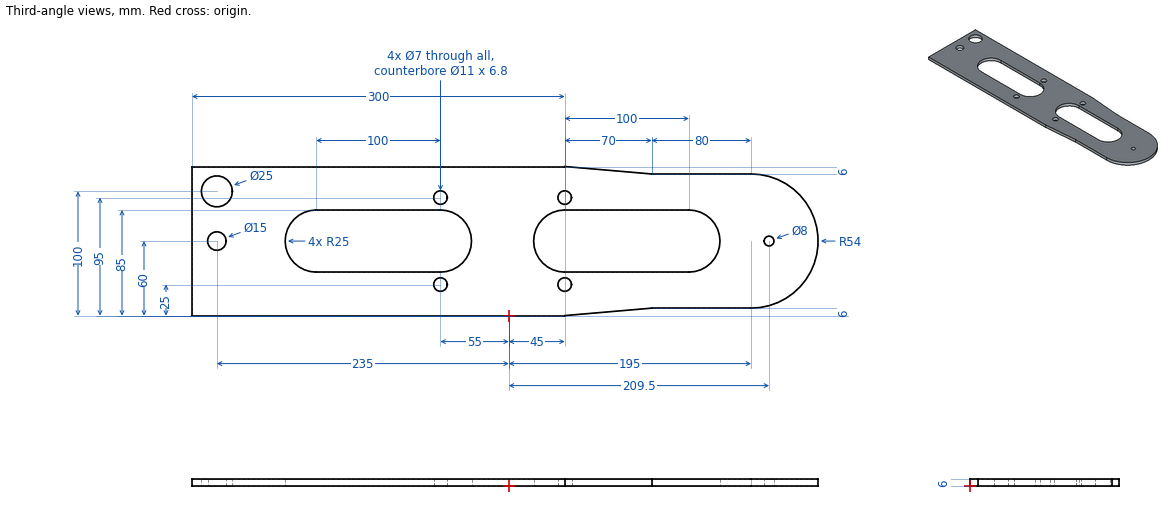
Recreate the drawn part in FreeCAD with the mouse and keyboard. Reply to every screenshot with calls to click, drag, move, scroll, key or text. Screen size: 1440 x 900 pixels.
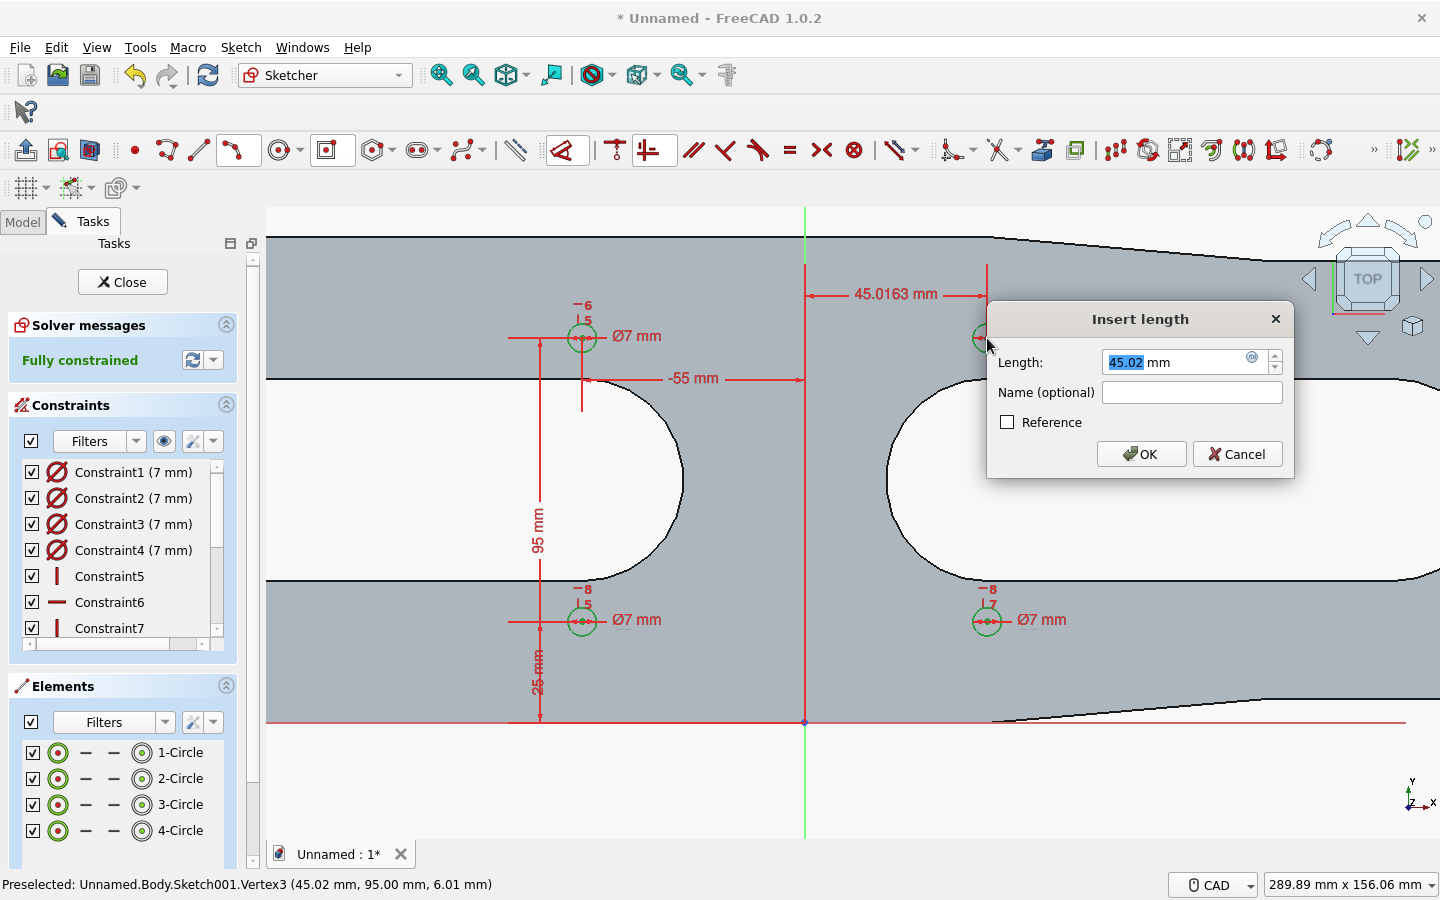
text(45)
key(Return)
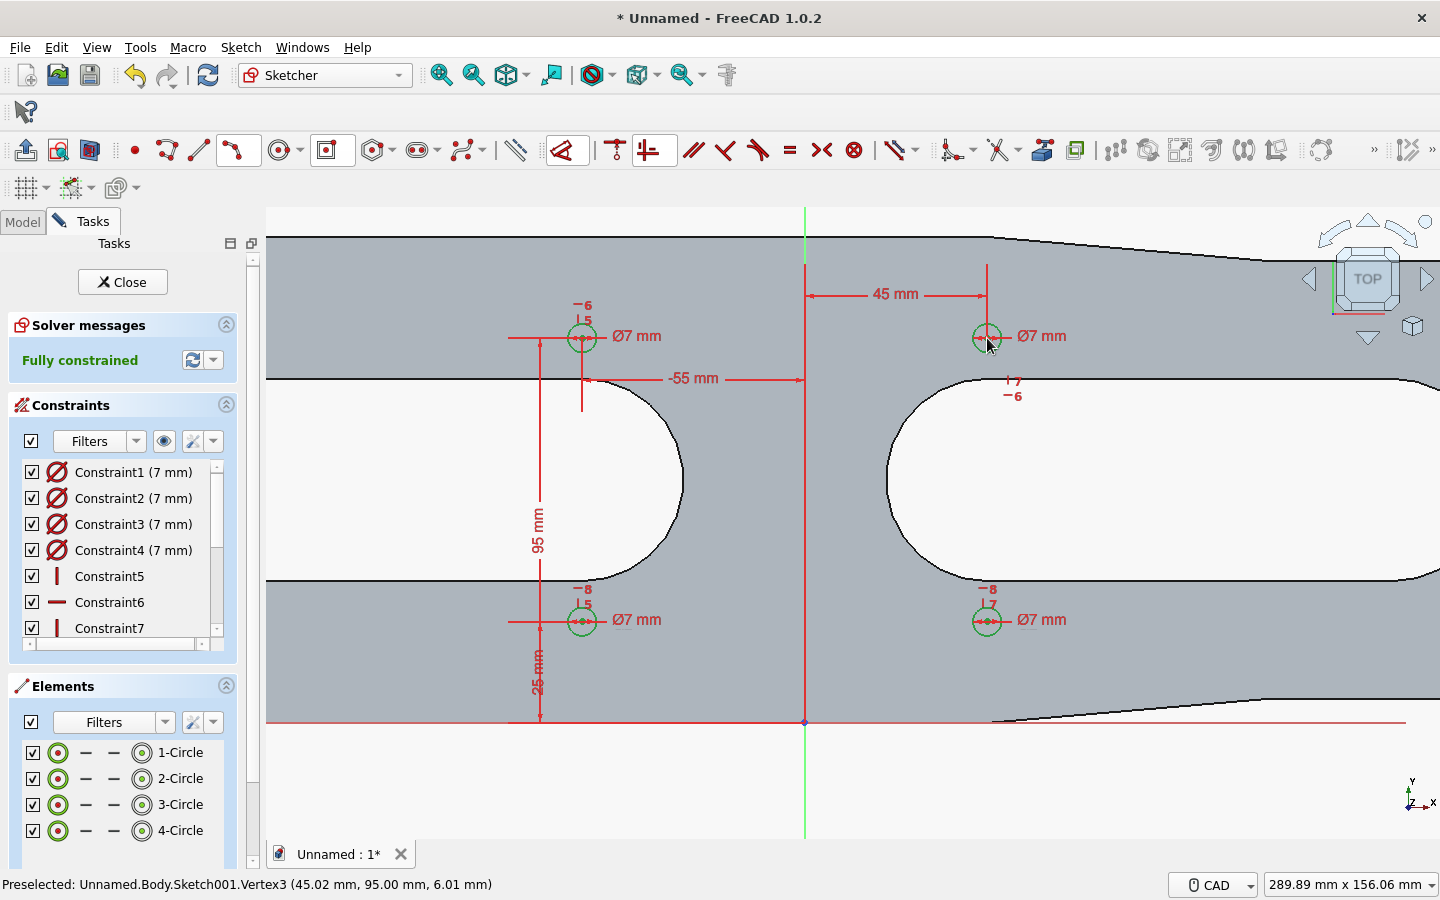
click(123, 282)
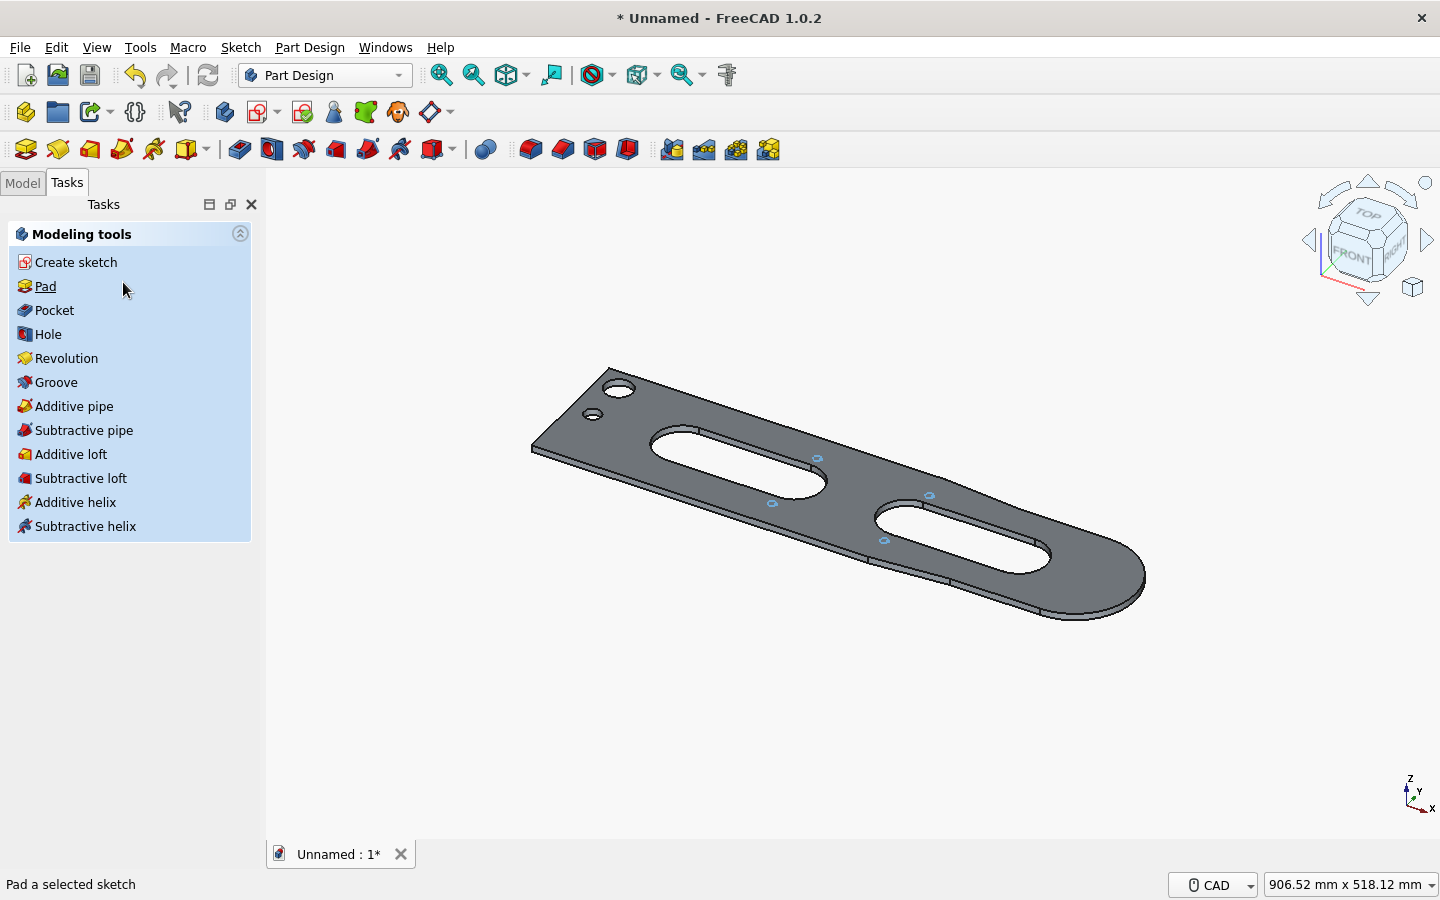
click(272, 150)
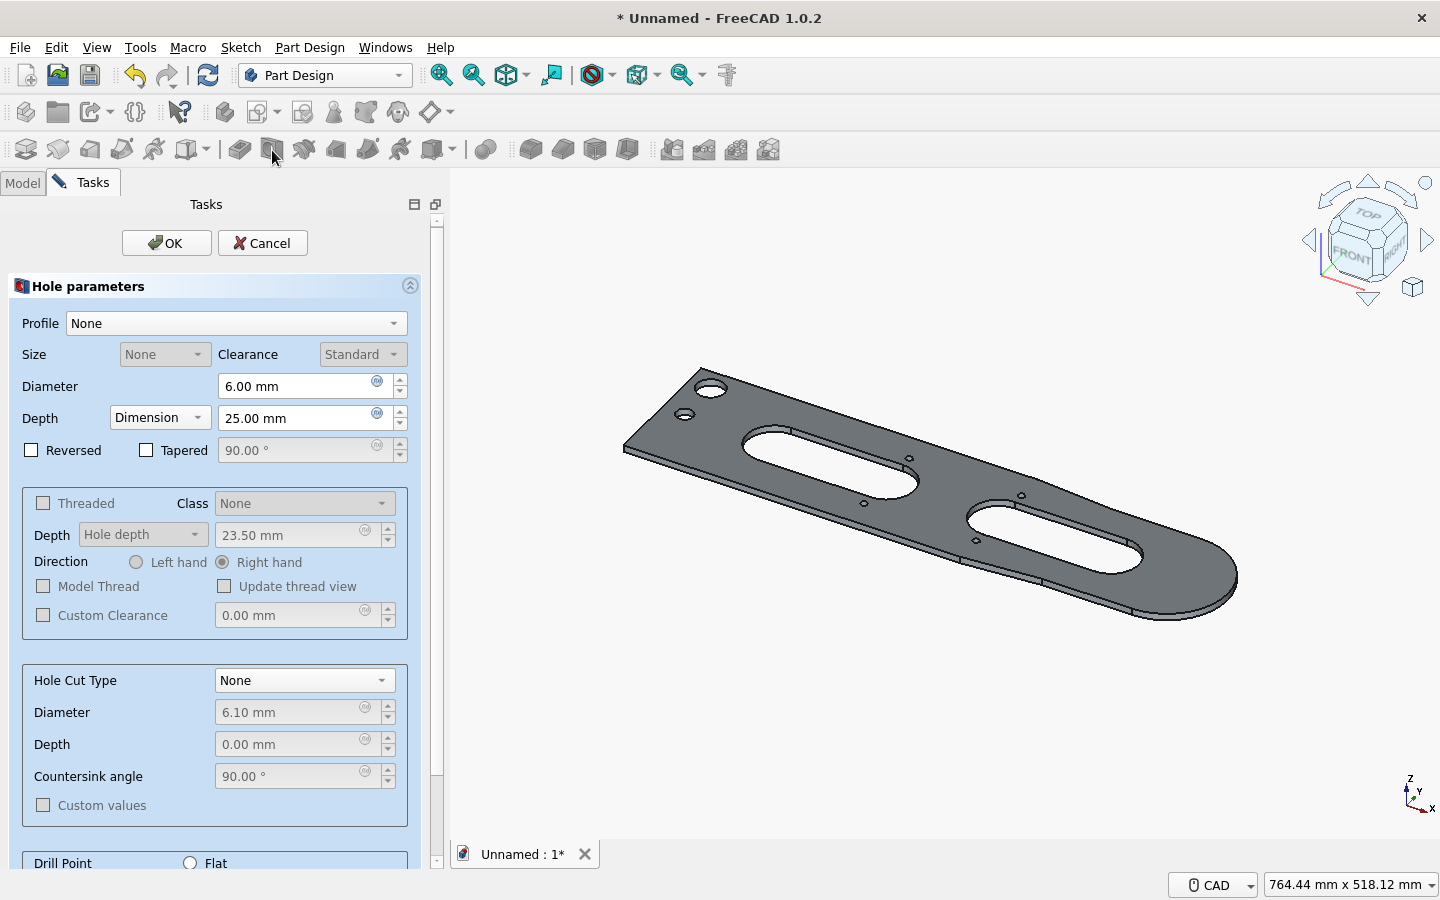
triple_click(305, 386)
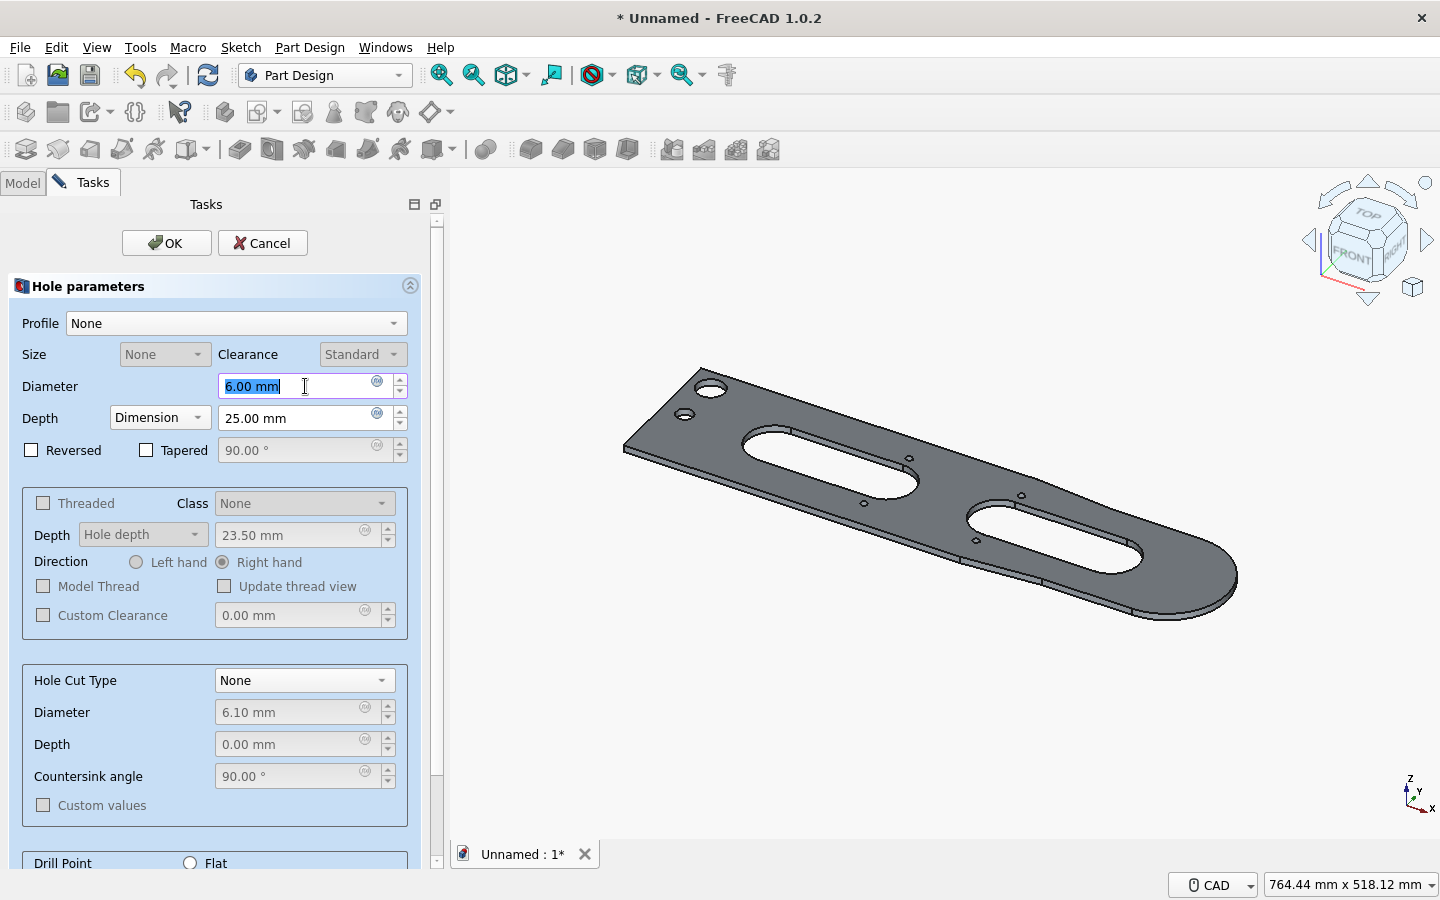
text(7)
key(Tab)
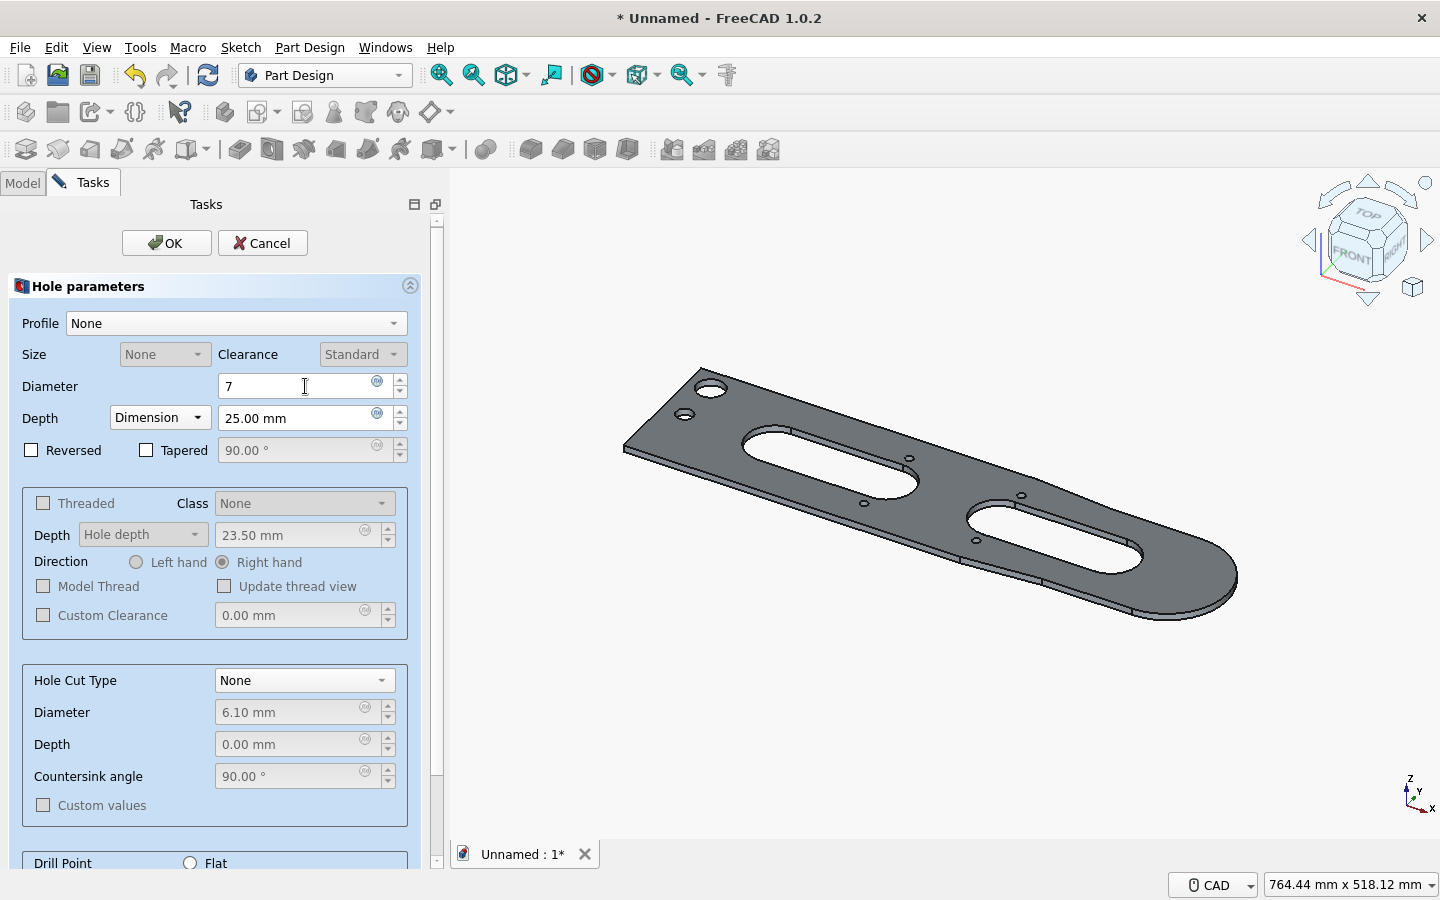
click(161, 418)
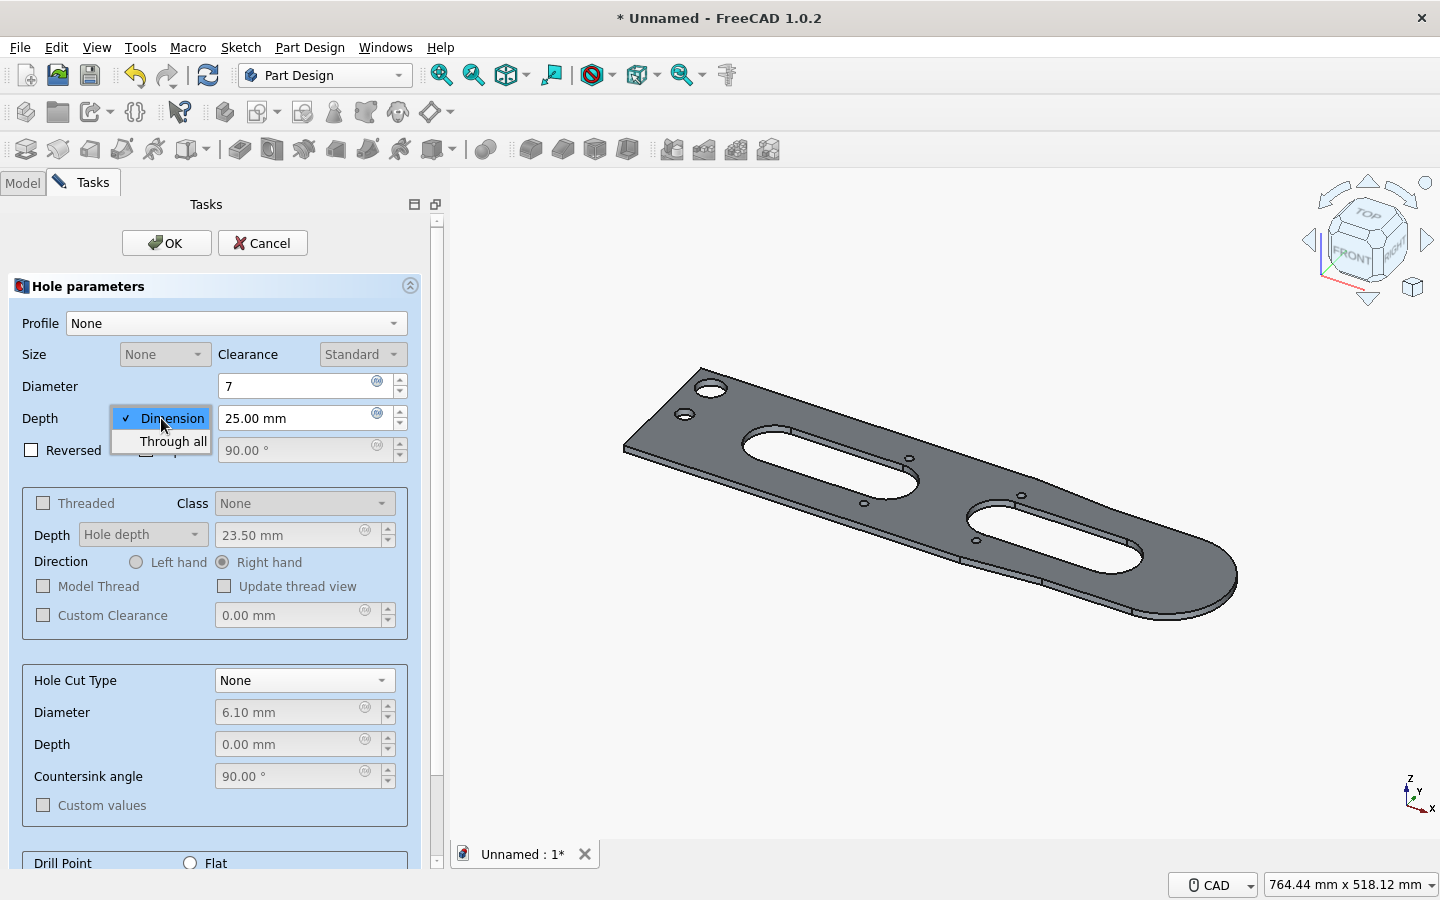
click(160, 442)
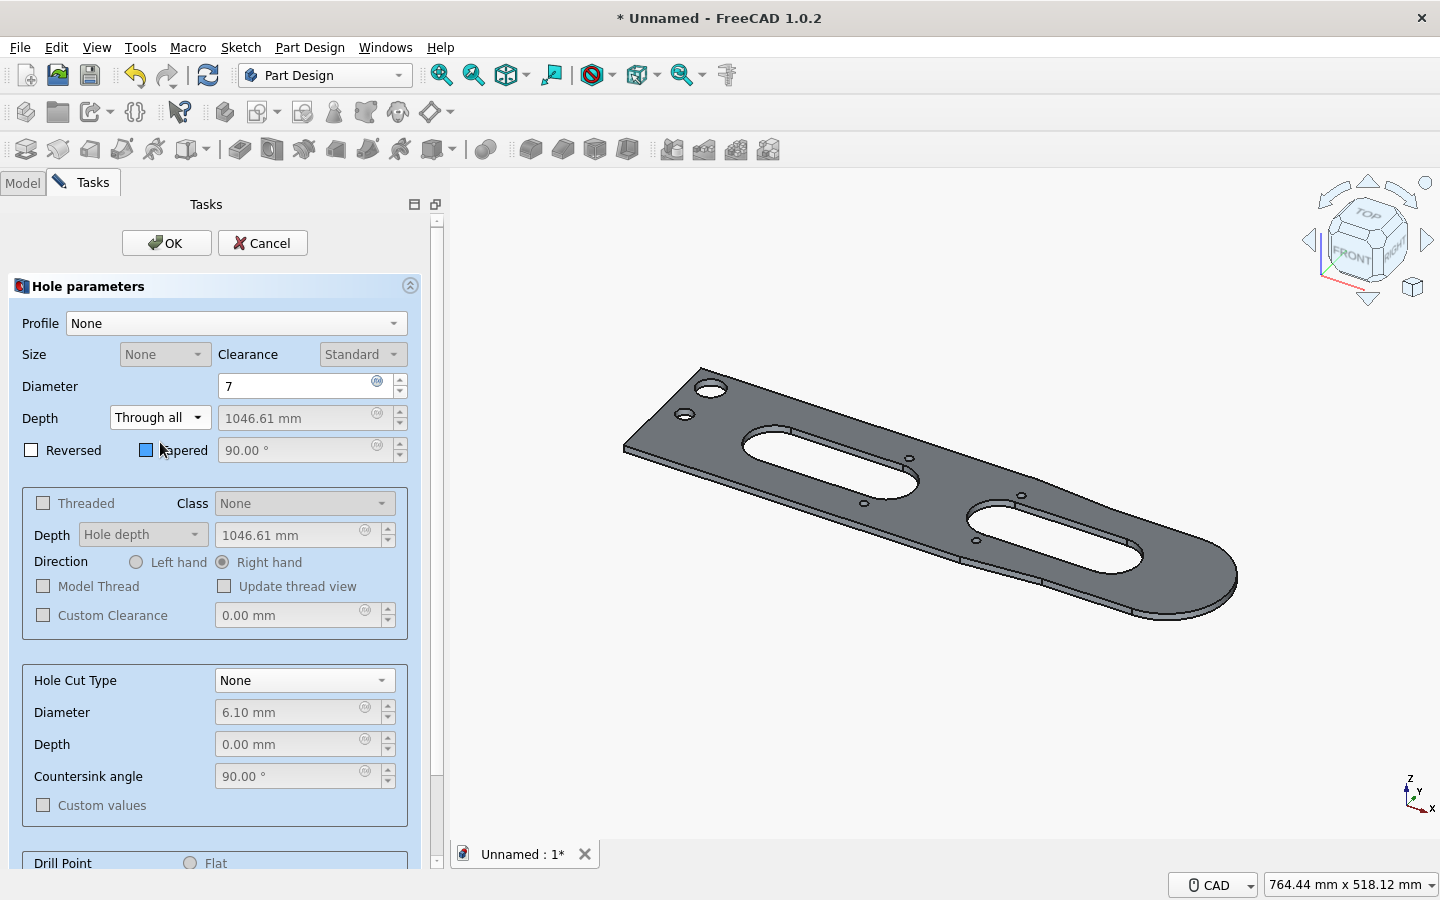
click(306, 680)